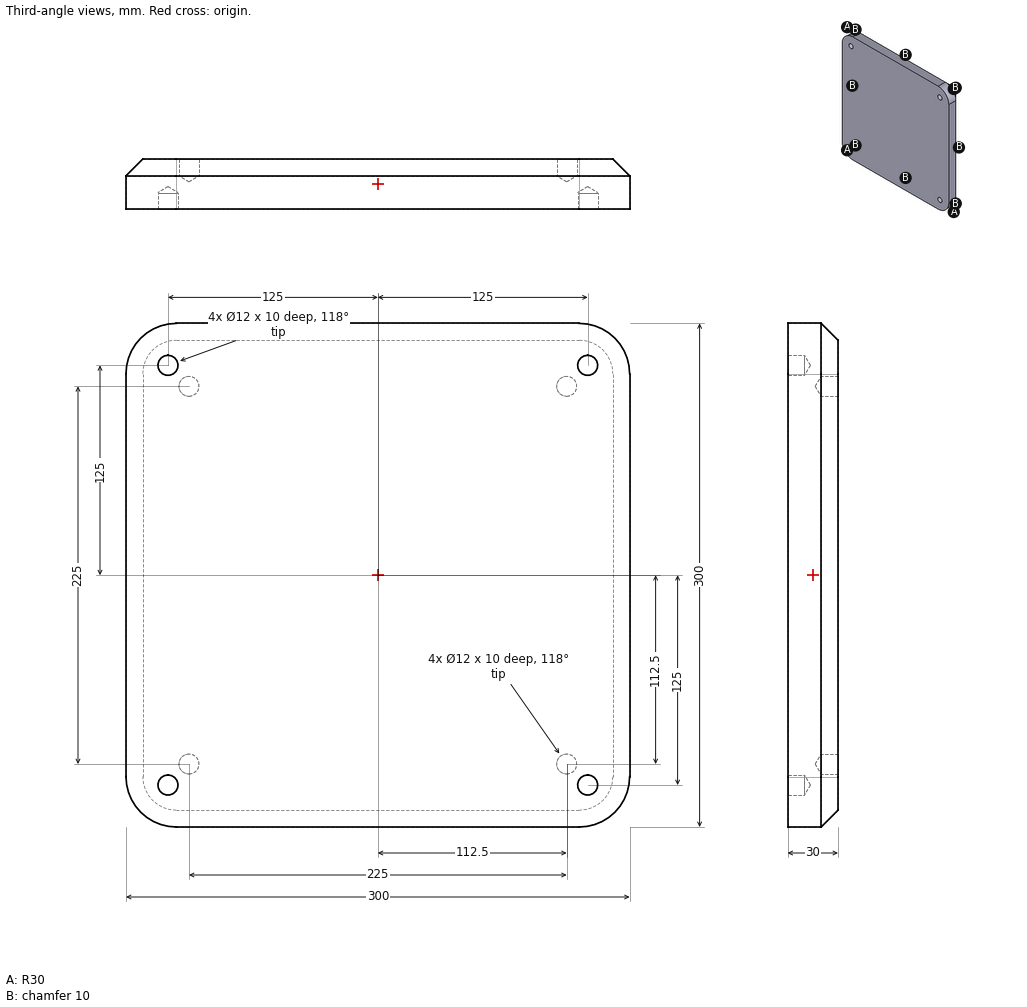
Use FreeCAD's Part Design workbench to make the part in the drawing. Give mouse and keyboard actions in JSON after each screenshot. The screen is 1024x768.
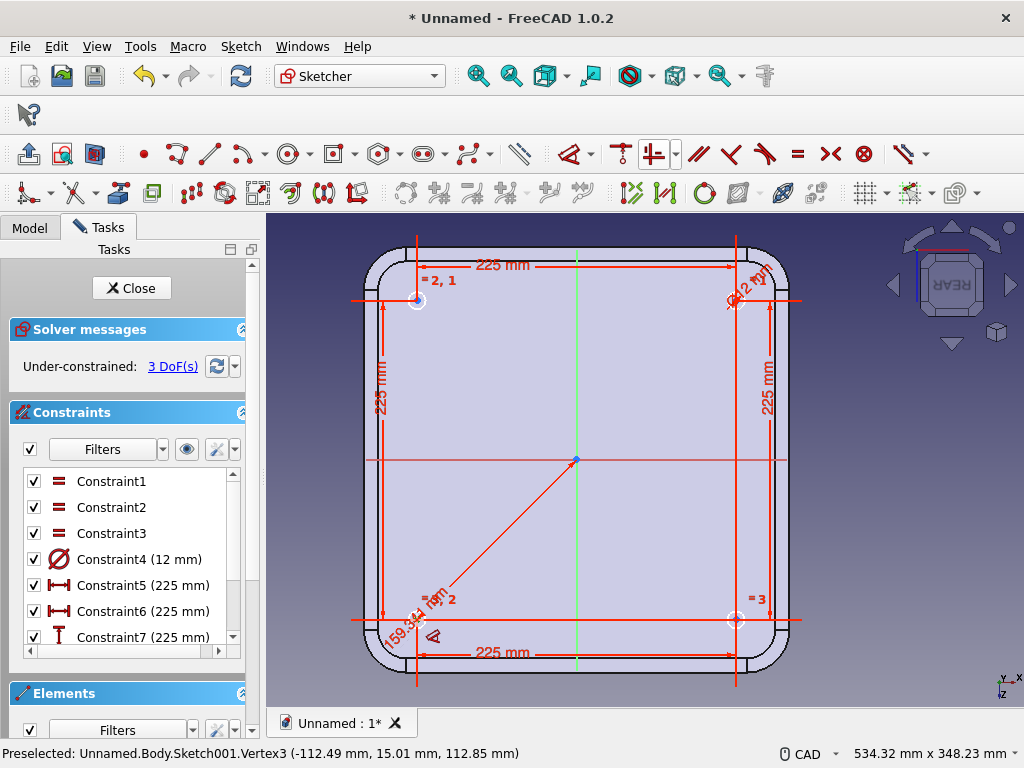
{"action": "left_click", "coordinate": [736, 620]}
{"action": "left_click", "coordinate": [650, 654]}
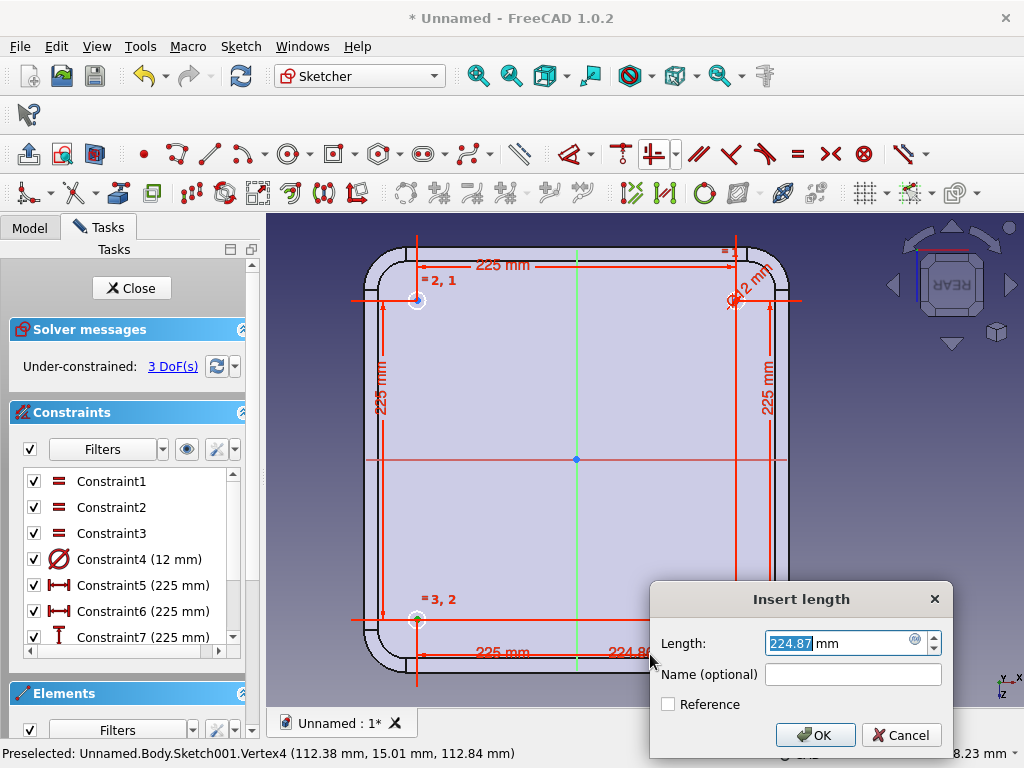
{"action": "type", "text": "225"}
{"action": "key", "text": "Return"}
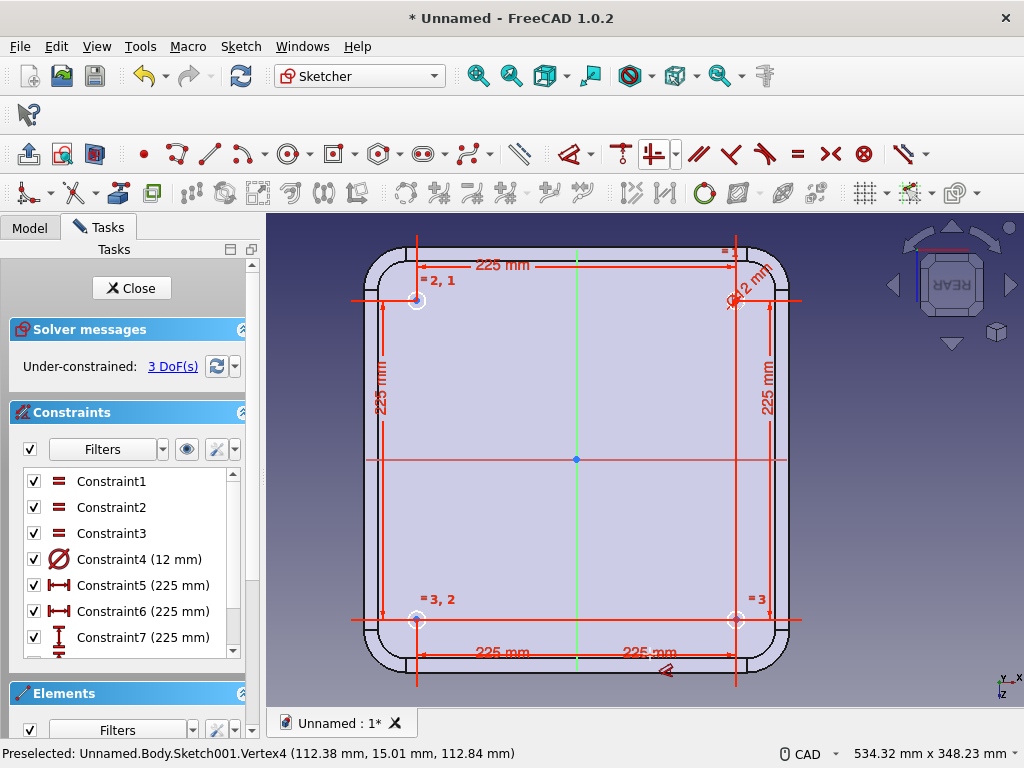
{"action": "left_click", "coordinate": [736, 301]}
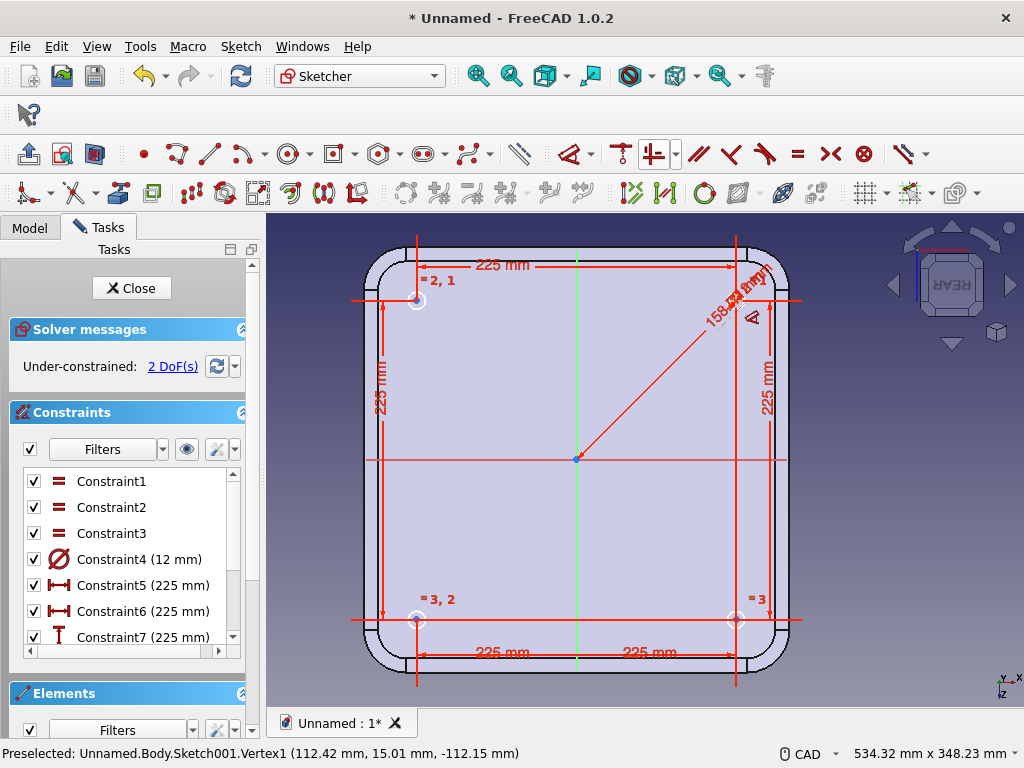
{"action": "left_click", "coordinate": [736, 620]}
{"action": "left_click", "coordinate": [770, 534]}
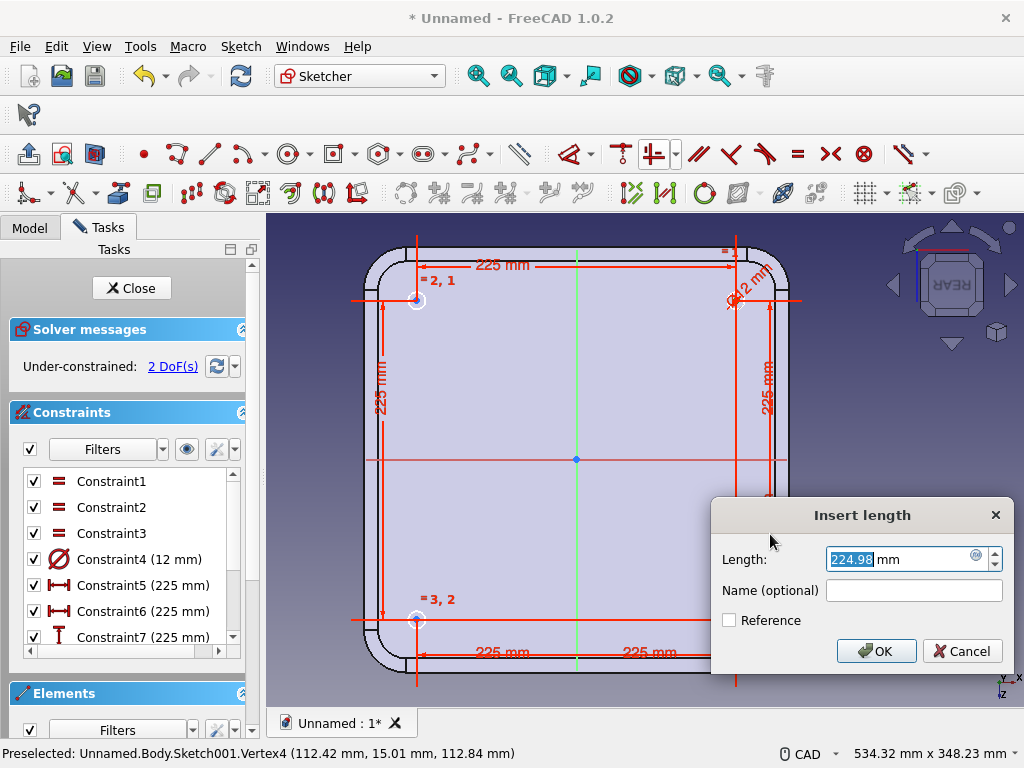
{"action": "type", "text": "225"}
{"action": "key", "text": "Return"}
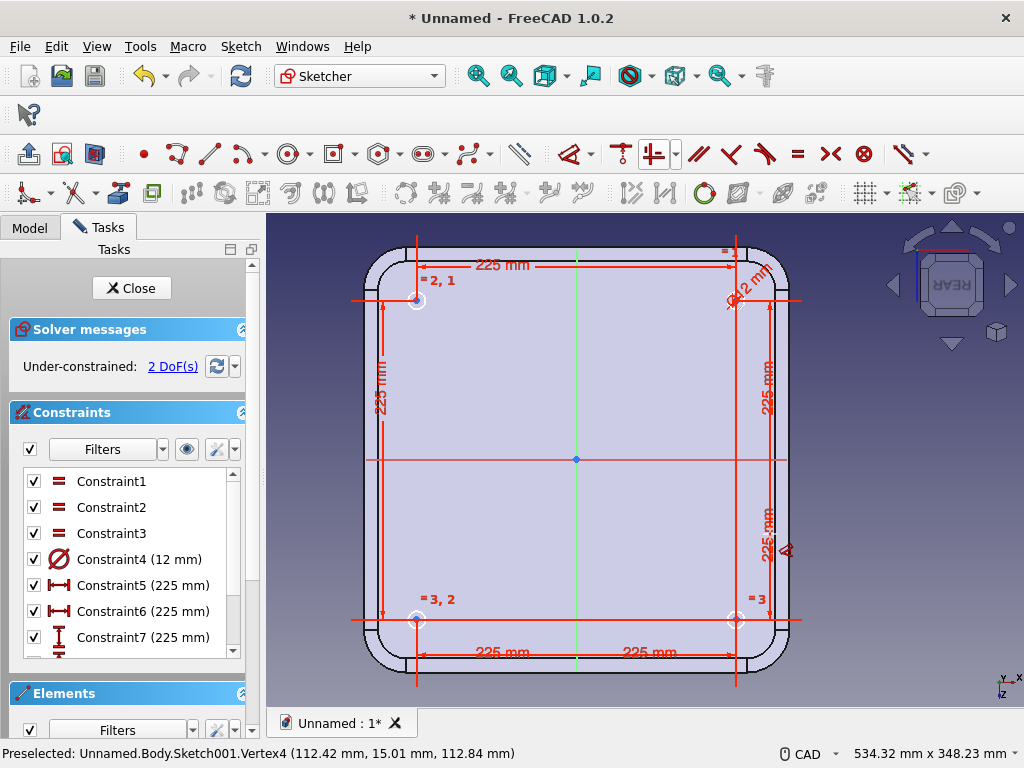
{"action": "left_click", "coordinate": [736, 301]}
{"action": "left_click", "coordinate": [656, 267]}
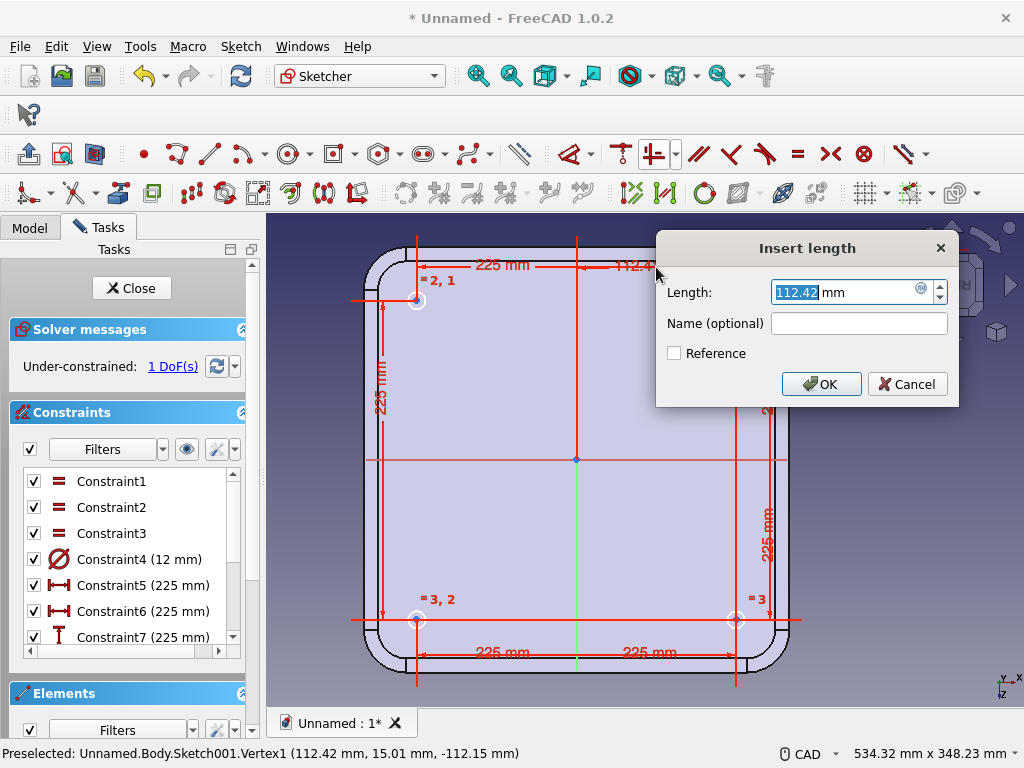
{"action": "type", "text": "112.5"}
{"action": "key", "text": "Return"}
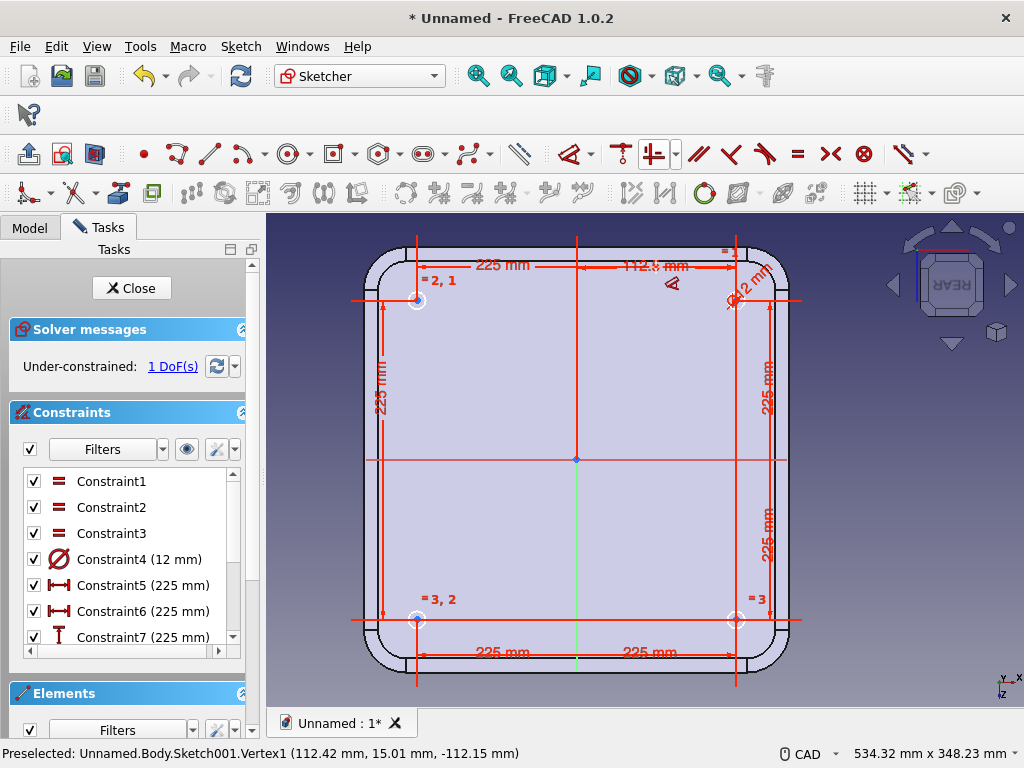
{"action": "left_click", "coordinate": [736, 301]}
{"action": "left_click", "coordinate": [770, 344]}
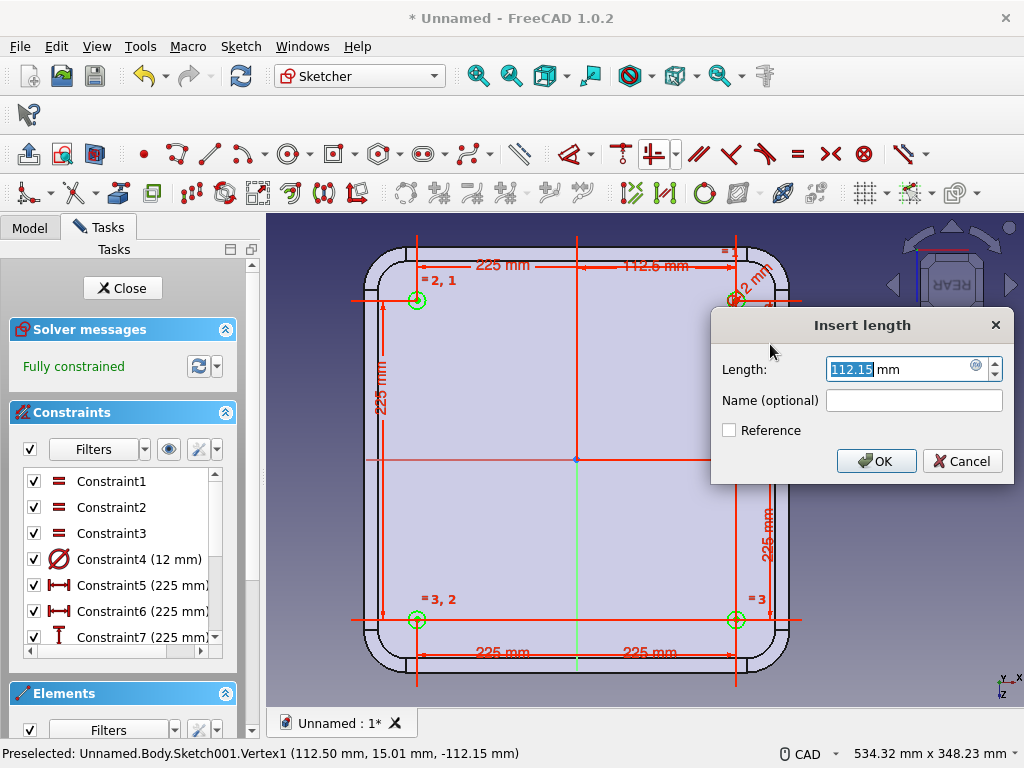
{"action": "type", "text": "112.5"}
{"action": "key", "text": "Return"}
{"action": "key", "text": "Escape"}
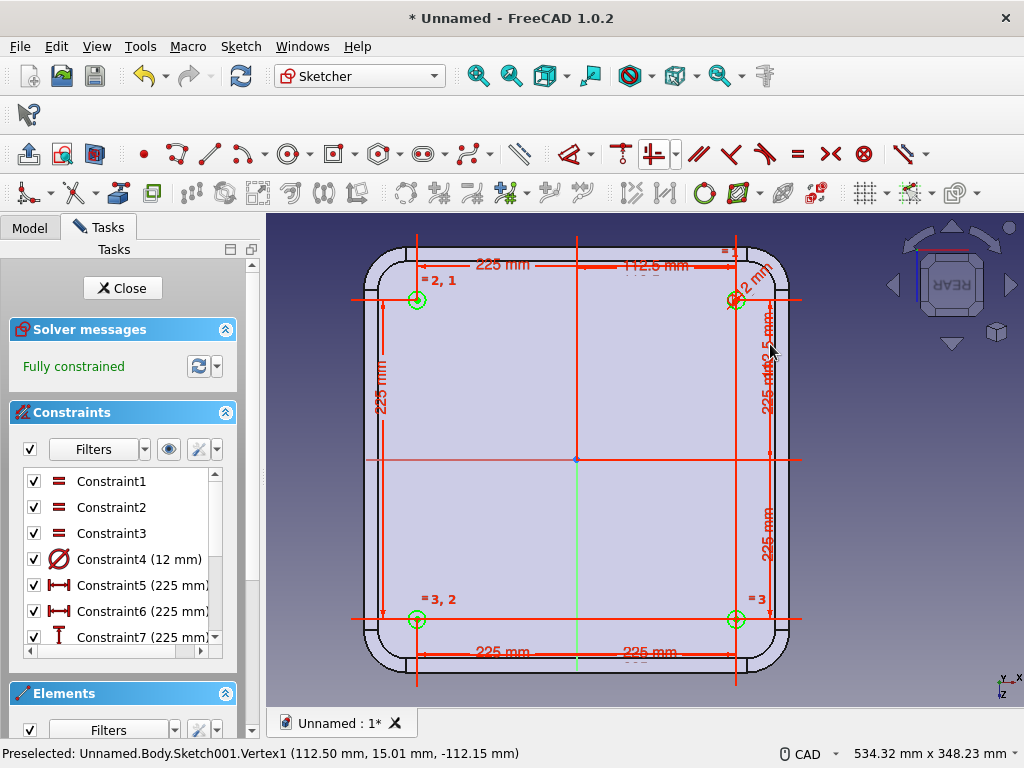
{"action": "left_click", "coordinate": [123, 288]}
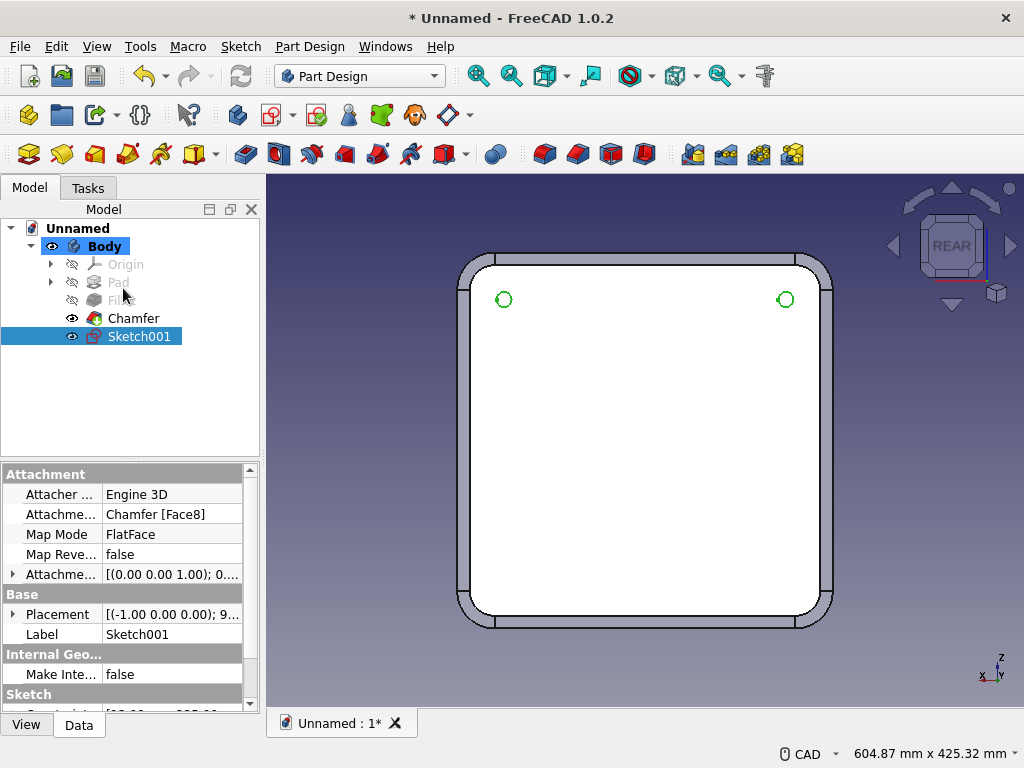
{"action": "left_click", "coordinate": [279, 154]}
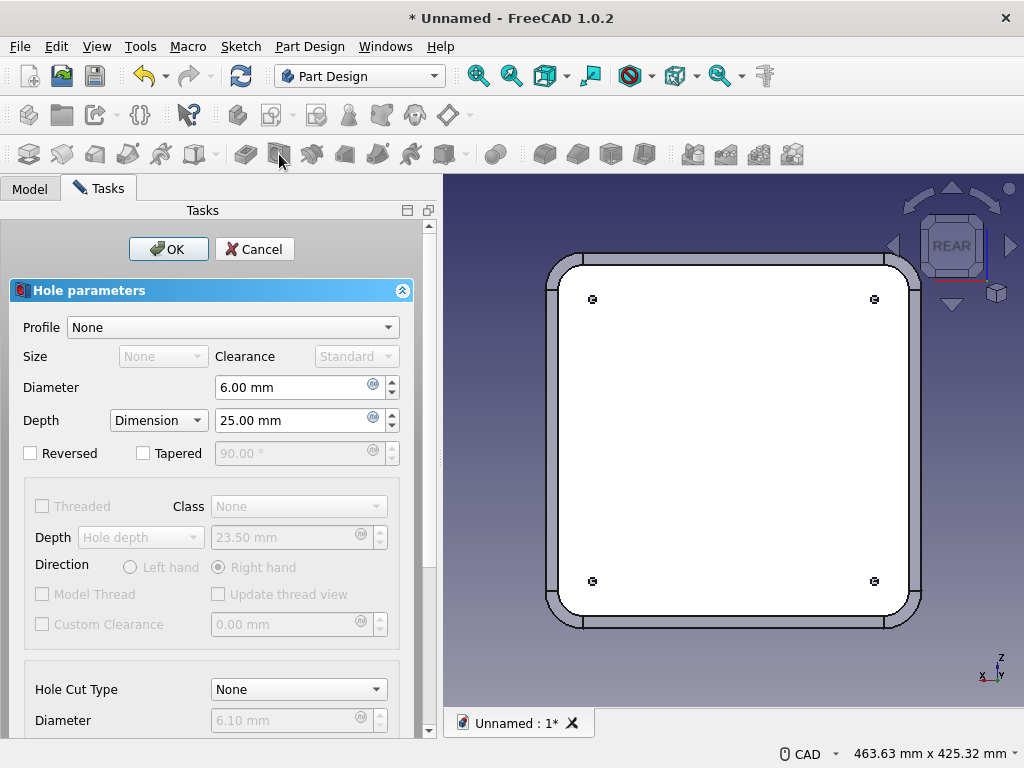
{"action": "triple_click", "coordinate": [300, 388]}